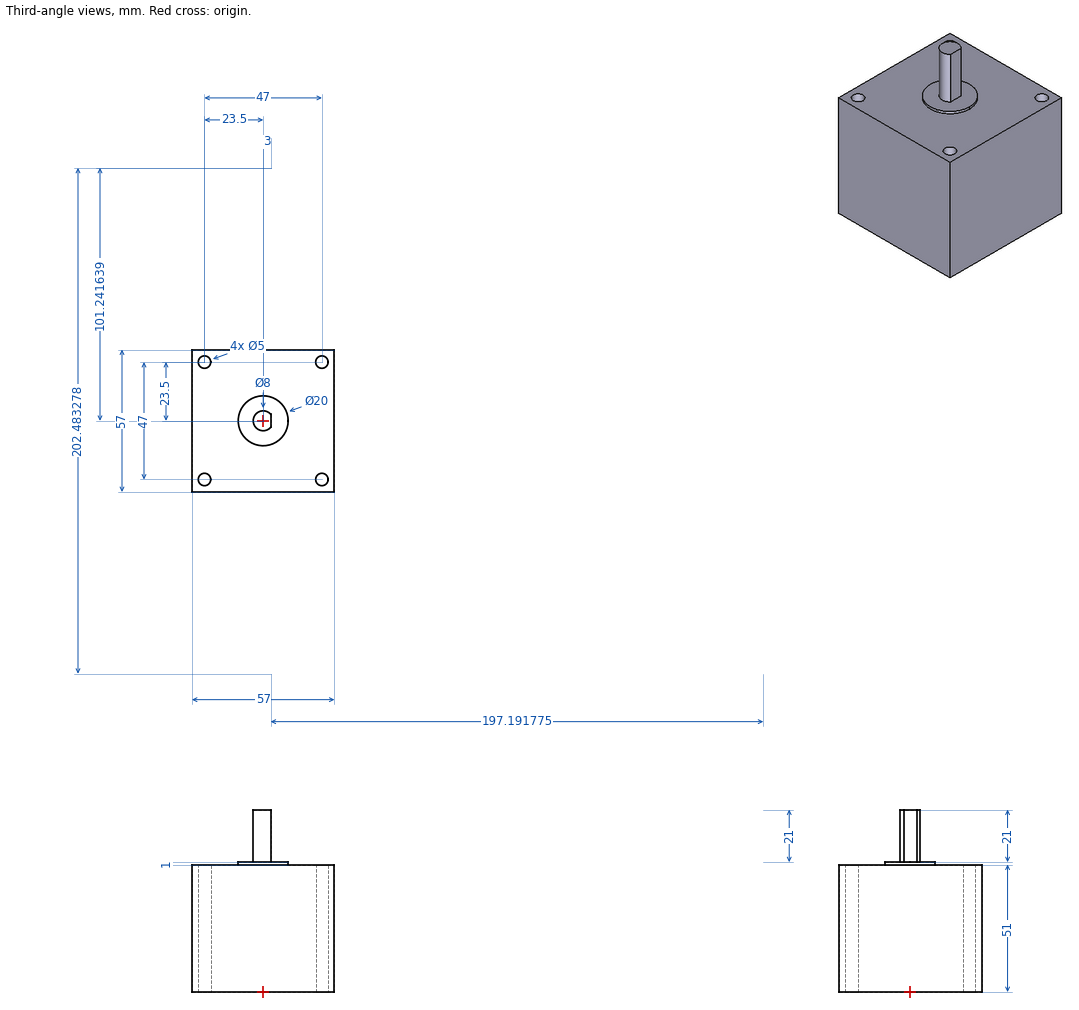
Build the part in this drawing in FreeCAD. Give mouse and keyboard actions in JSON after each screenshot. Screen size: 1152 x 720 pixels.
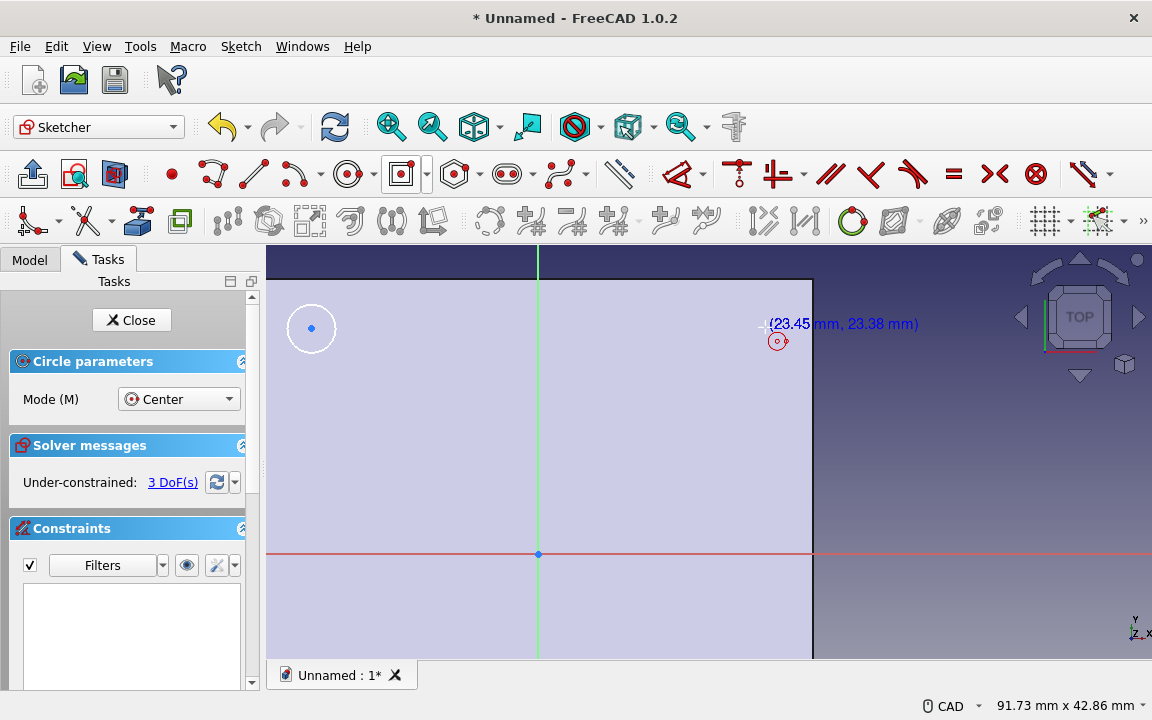
{"action": "left_click", "coordinate": [765, 327]}
{"action": "left_click", "coordinate": [782, 310]}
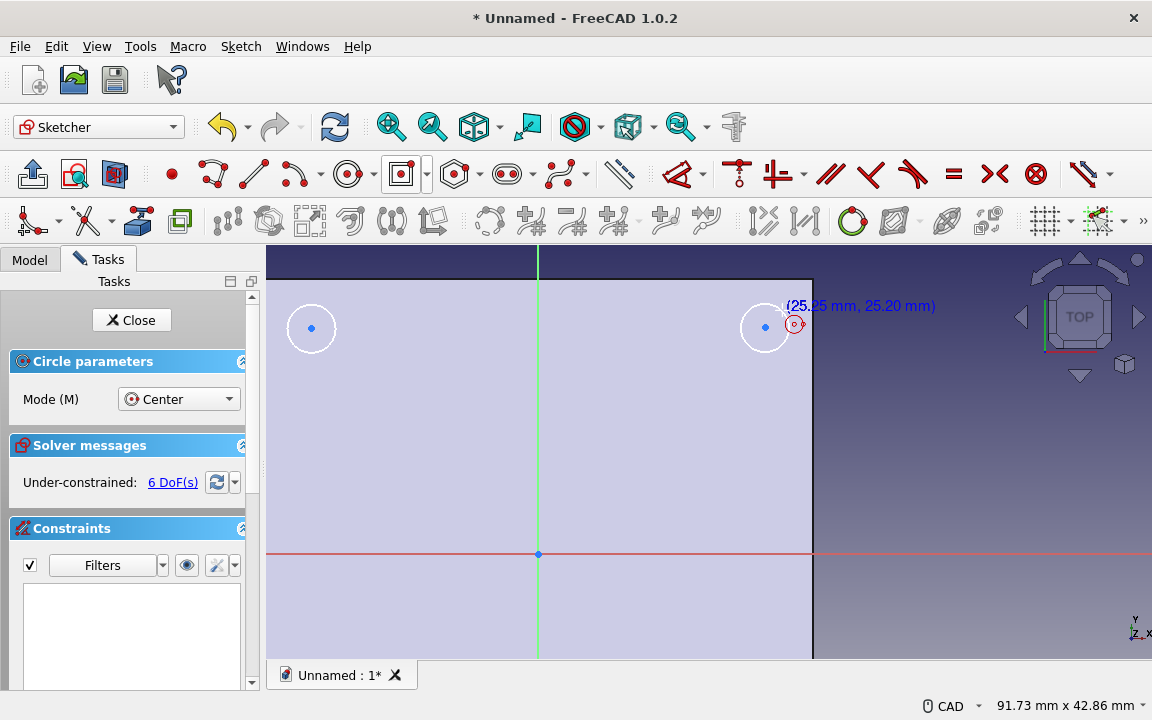
{"action": "scroll", "coordinate": [765, 327], "scroll_direction": "down", "scroll_amount": 3}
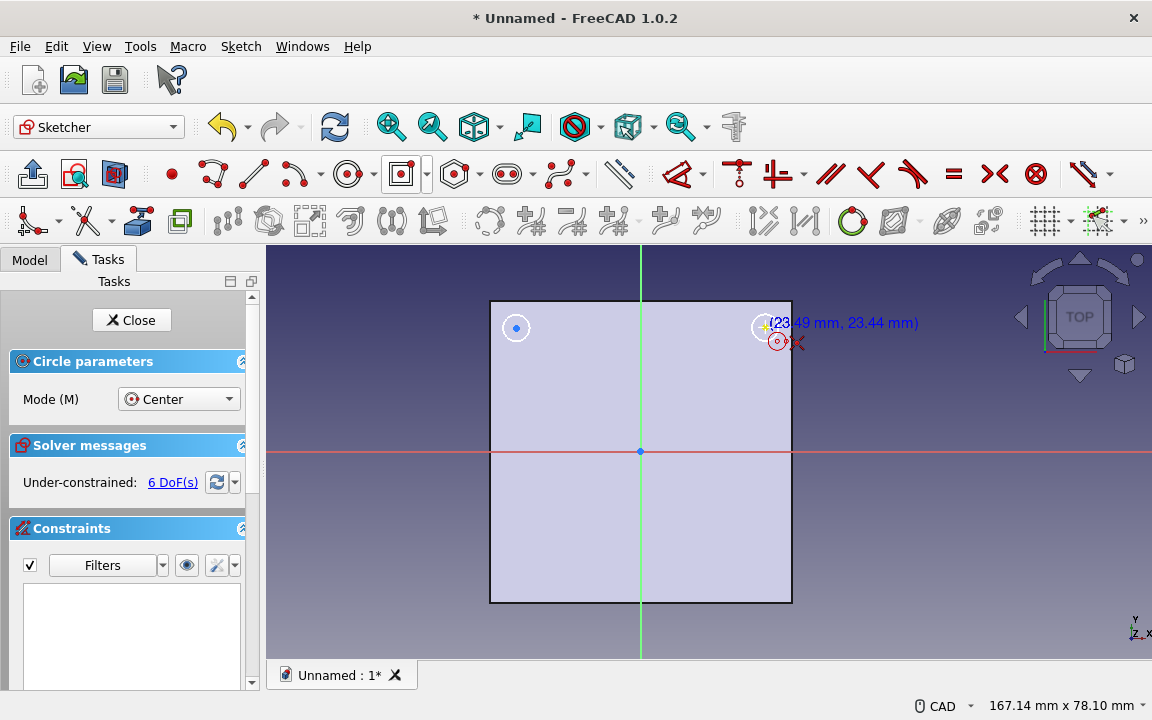
{"action": "scroll", "coordinate": [765, 576], "scroll_direction": "up", "scroll_amount": 3}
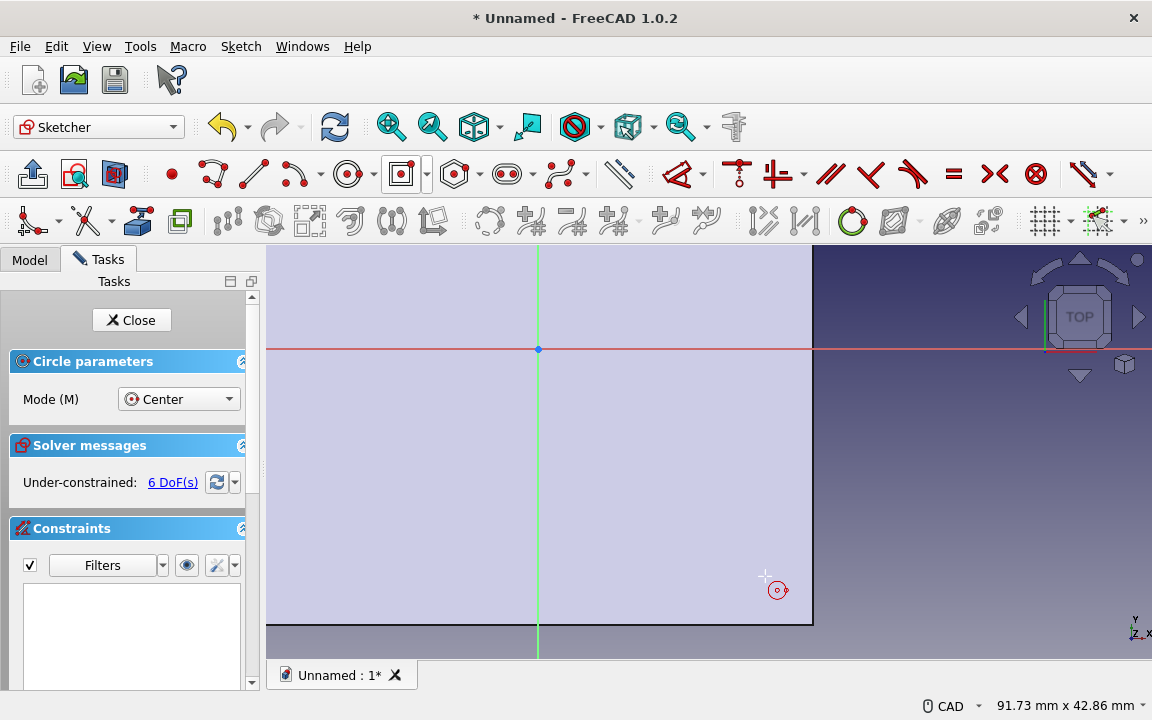
{"action": "left_click", "coordinate": [765, 576]}
{"action": "left_click", "coordinate": [782, 559]}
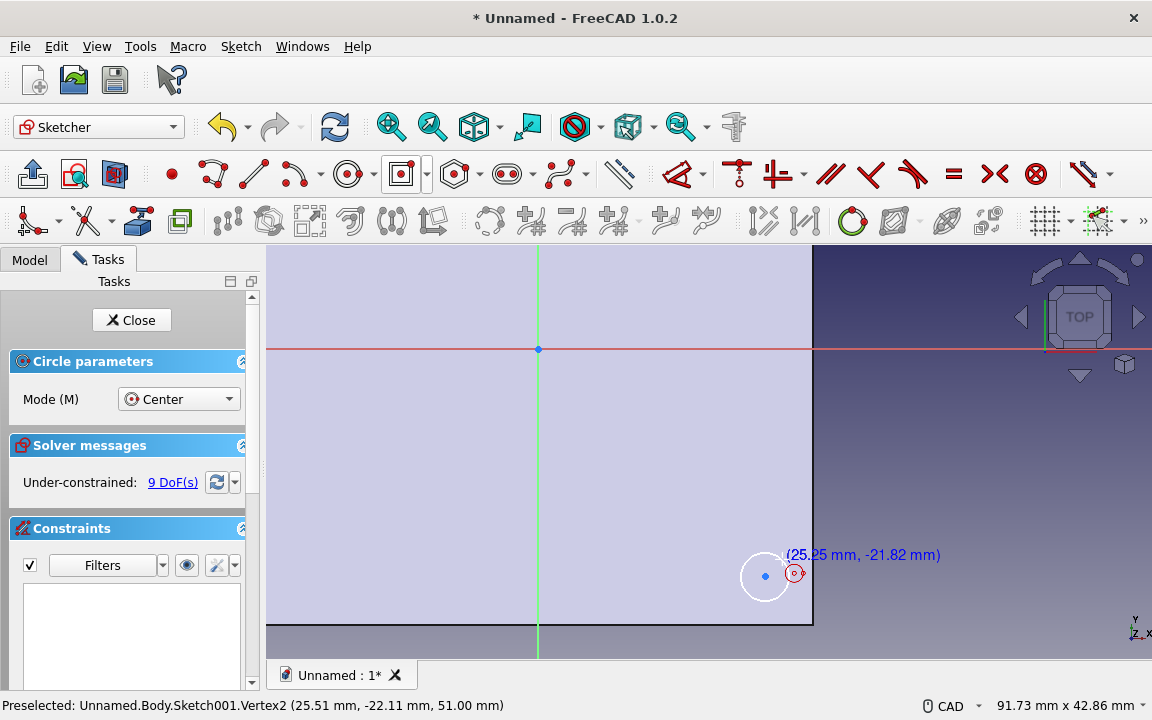
{"action": "left_click", "coordinate": [311, 576]}
{"action": "left_click", "coordinate": [328, 559]}
{"action": "key", "text": "Escape"}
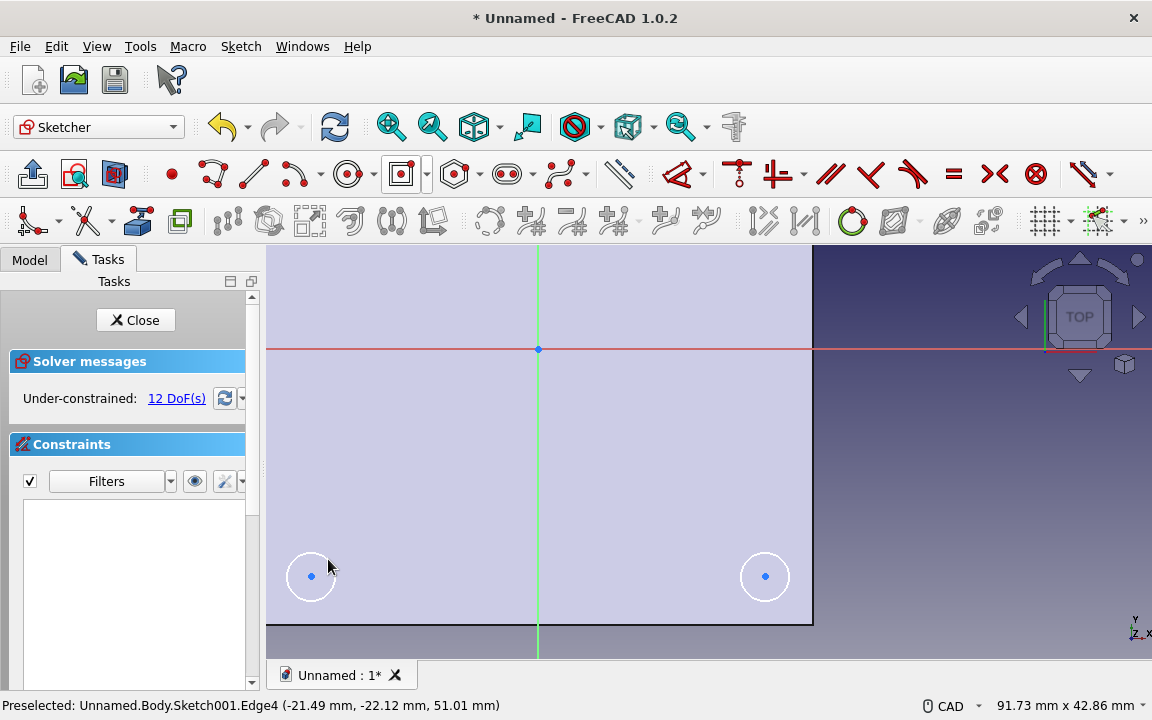
{"action": "scroll", "coordinate": [765, 577], "scroll_direction": "down", "scroll_amount": 3}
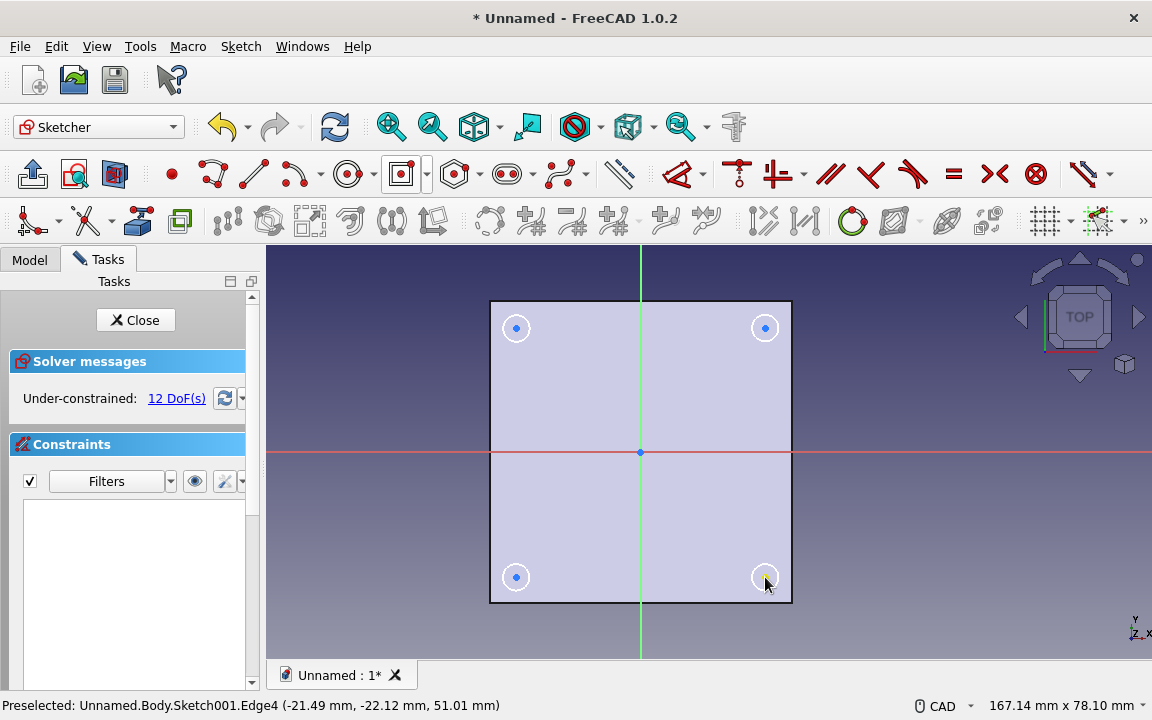
{"action": "left_click", "coordinate": [526, 319]}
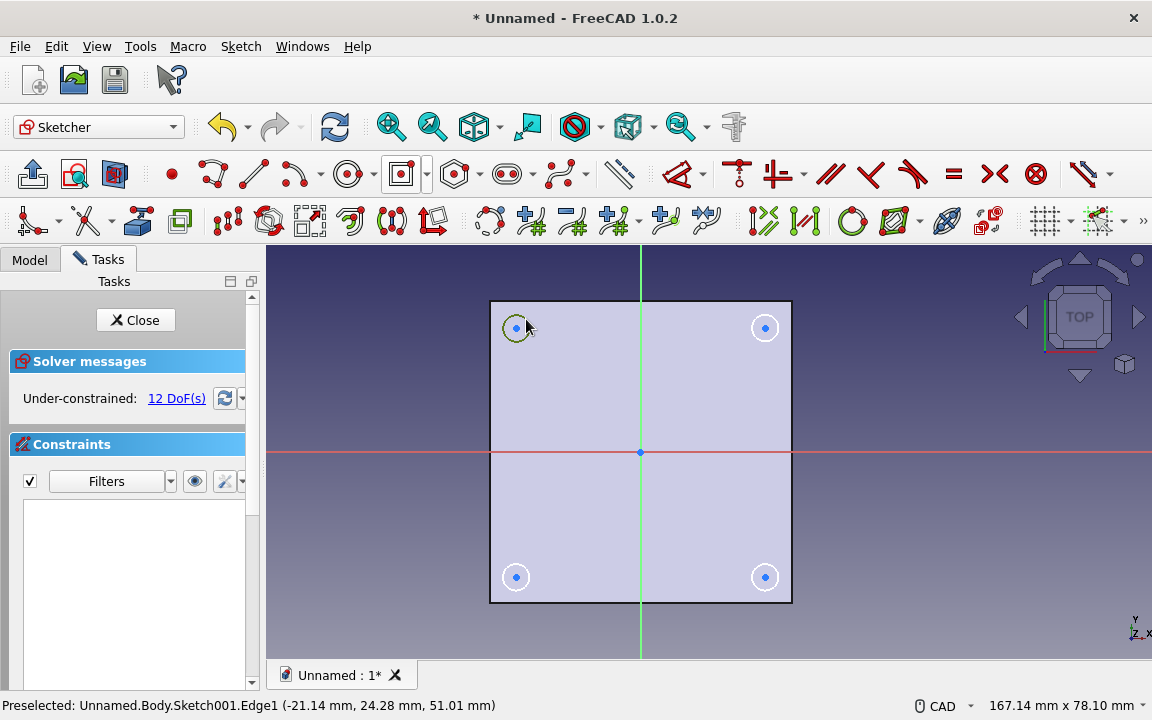
{"action": "left_click", "coordinate": [775, 319]}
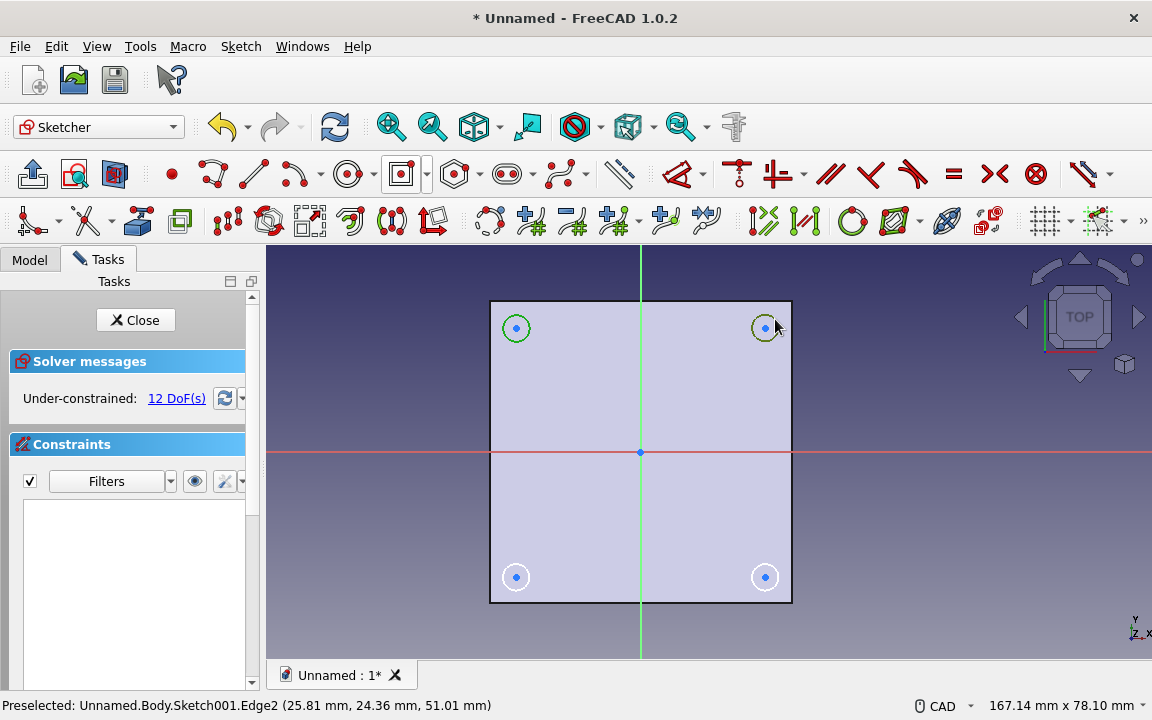
{"action": "left_click", "coordinate": [775, 568]}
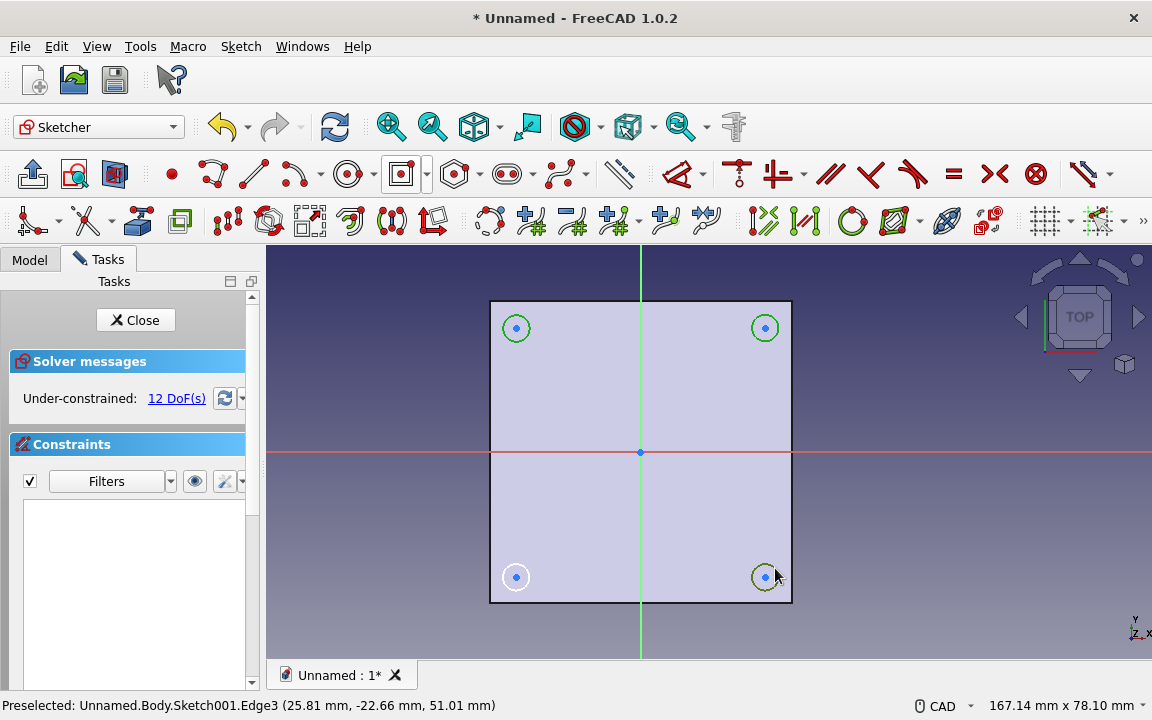
{"action": "left_click", "coordinate": [525, 568]}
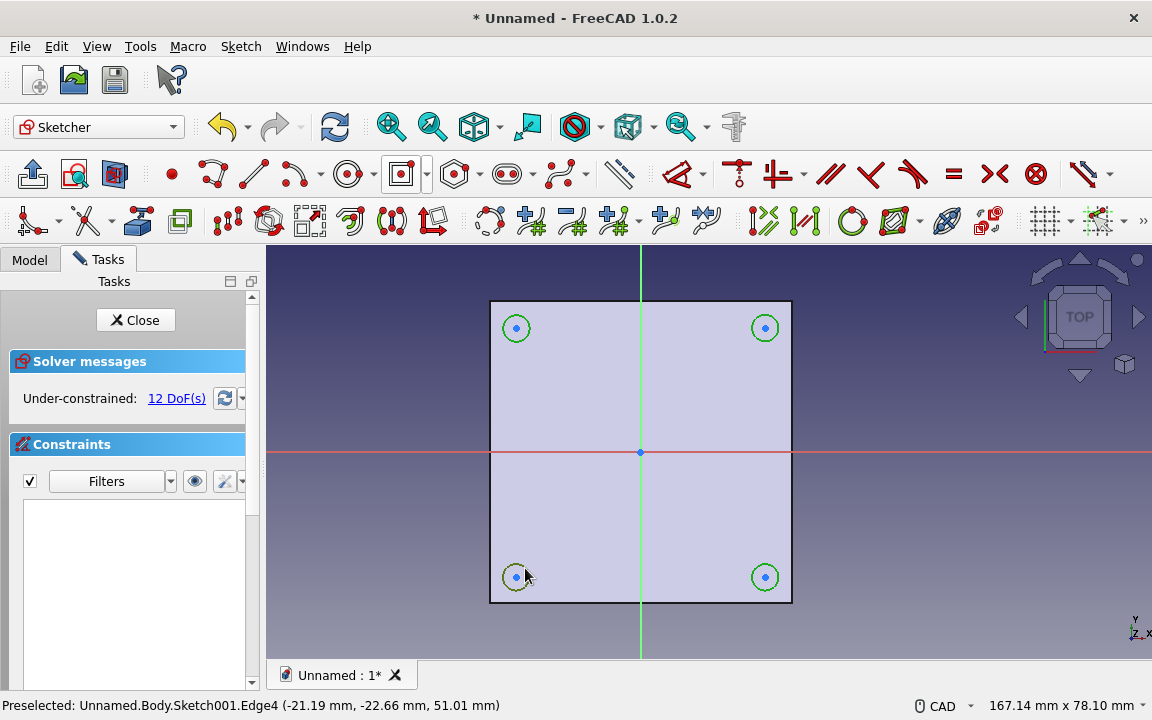
{"action": "left_click", "coordinate": [954, 174]}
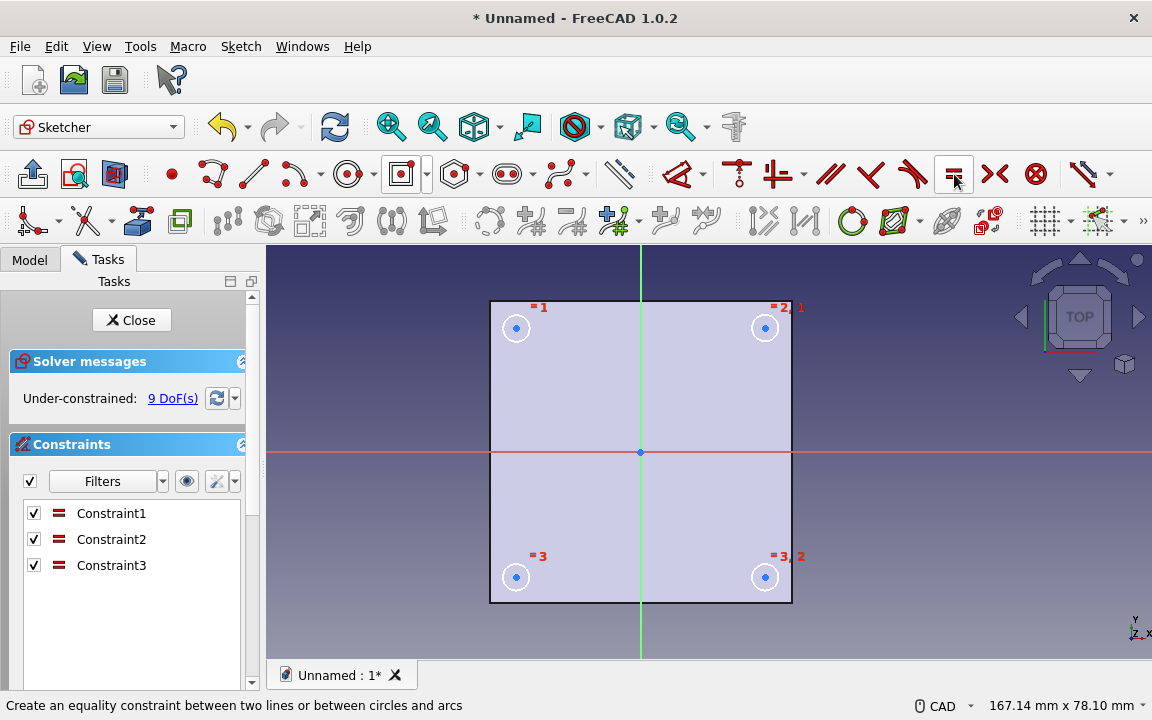
{"action": "left_click", "coordinate": [516, 329]}